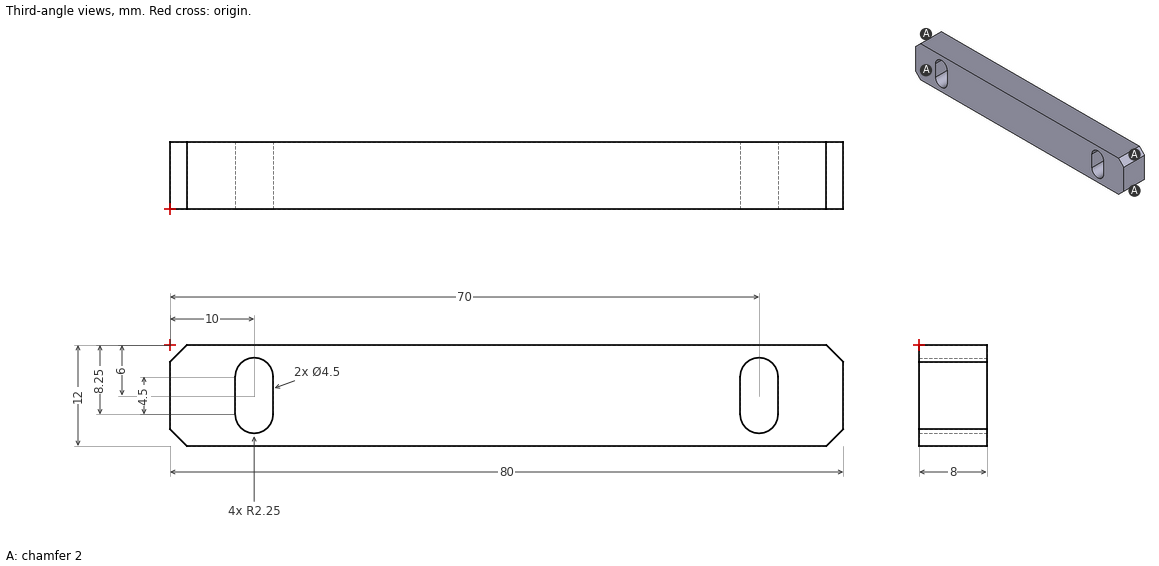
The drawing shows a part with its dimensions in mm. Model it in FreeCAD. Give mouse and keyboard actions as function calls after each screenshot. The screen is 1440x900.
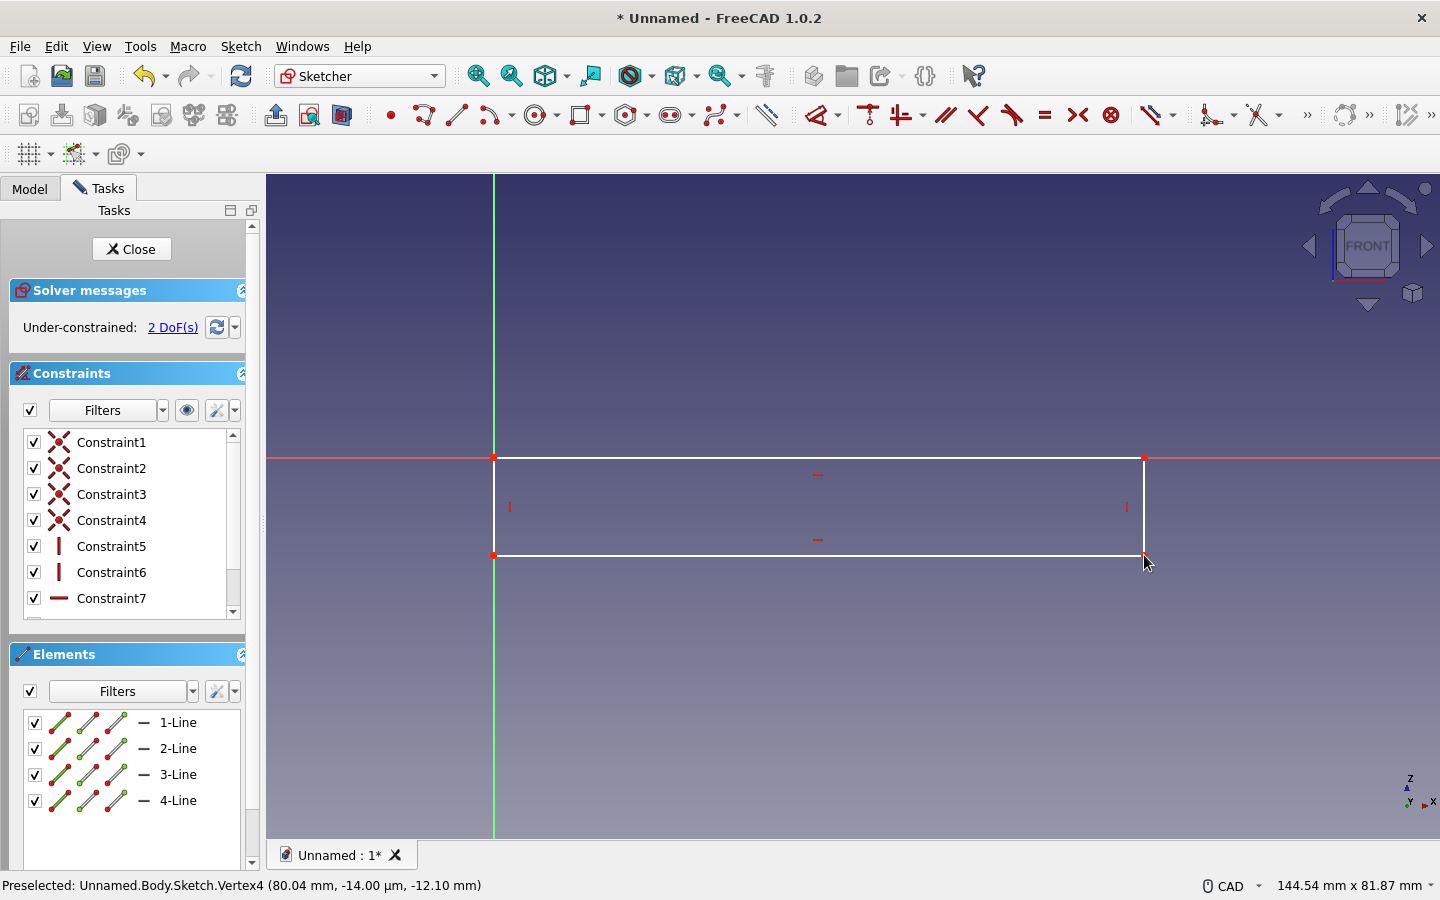
key(d)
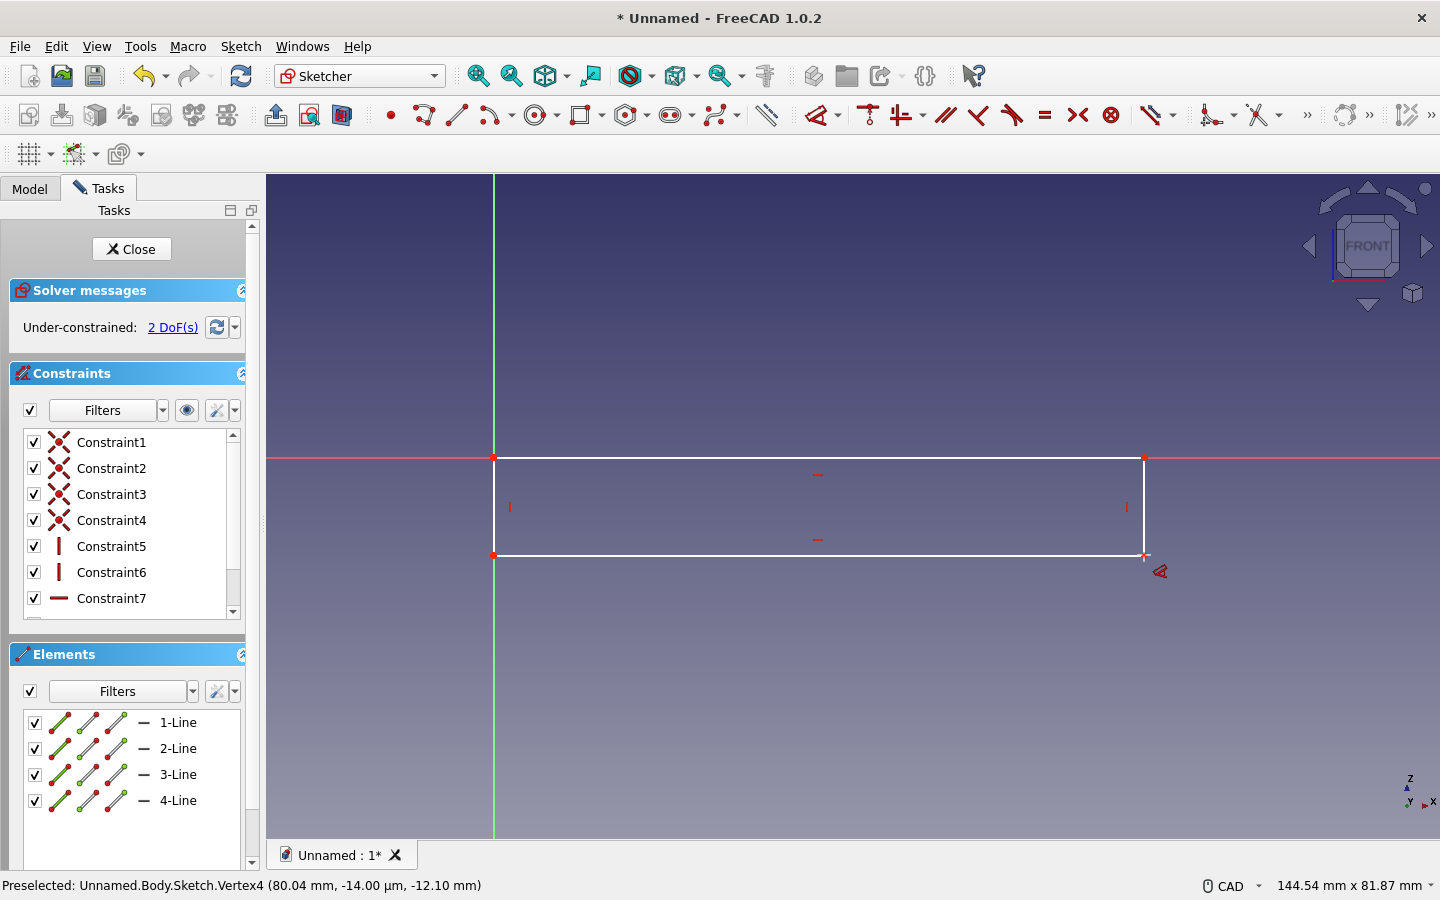
click(494, 487)
click(460, 507)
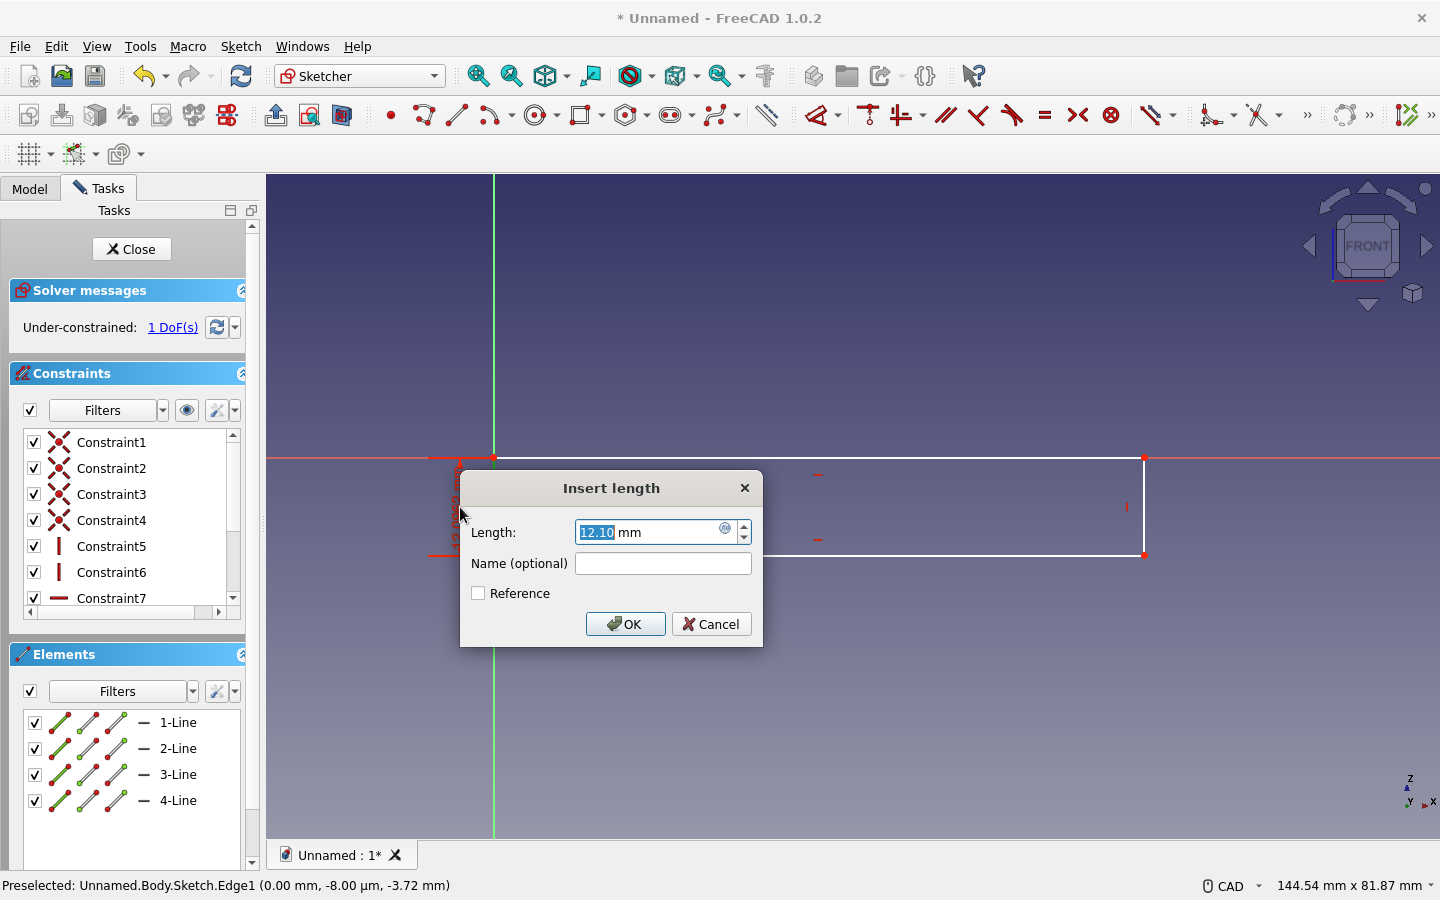
text(12)
key(Return)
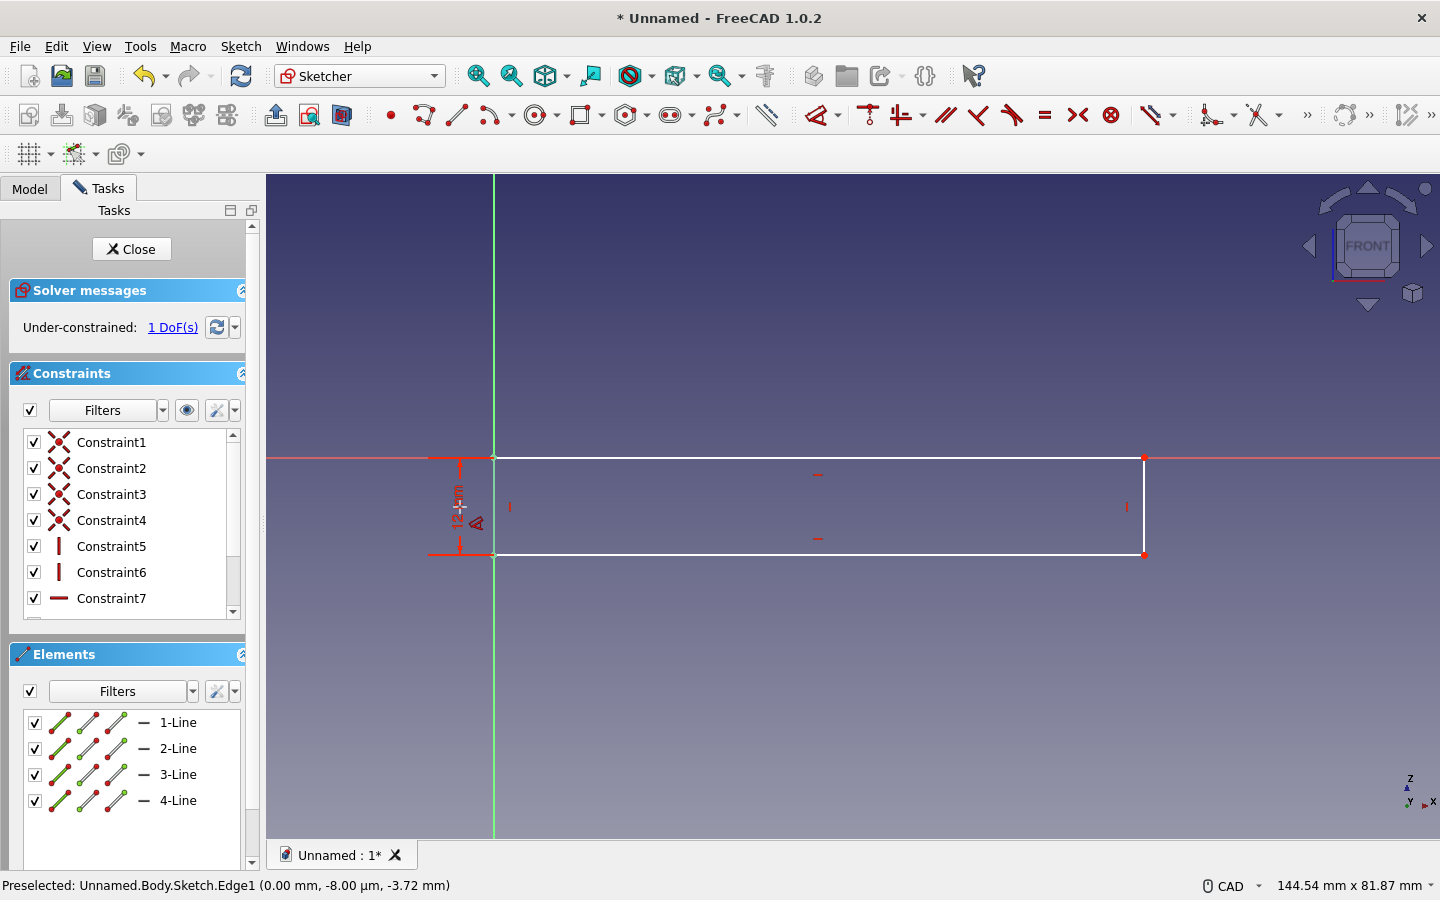
click(689, 555)
click(819, 589)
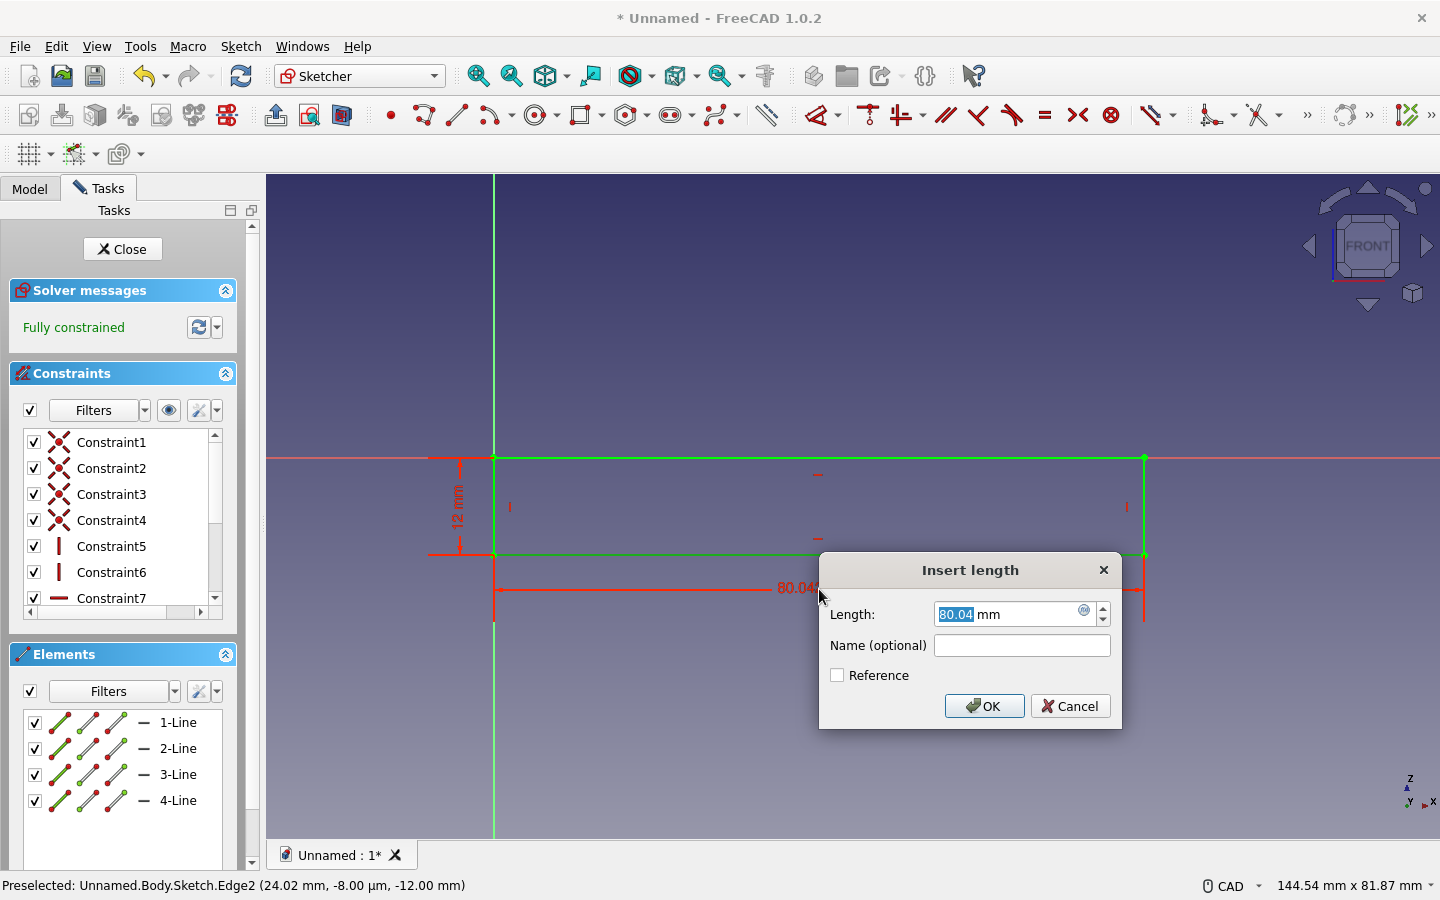
text(80)
key(Return)
key(Escape)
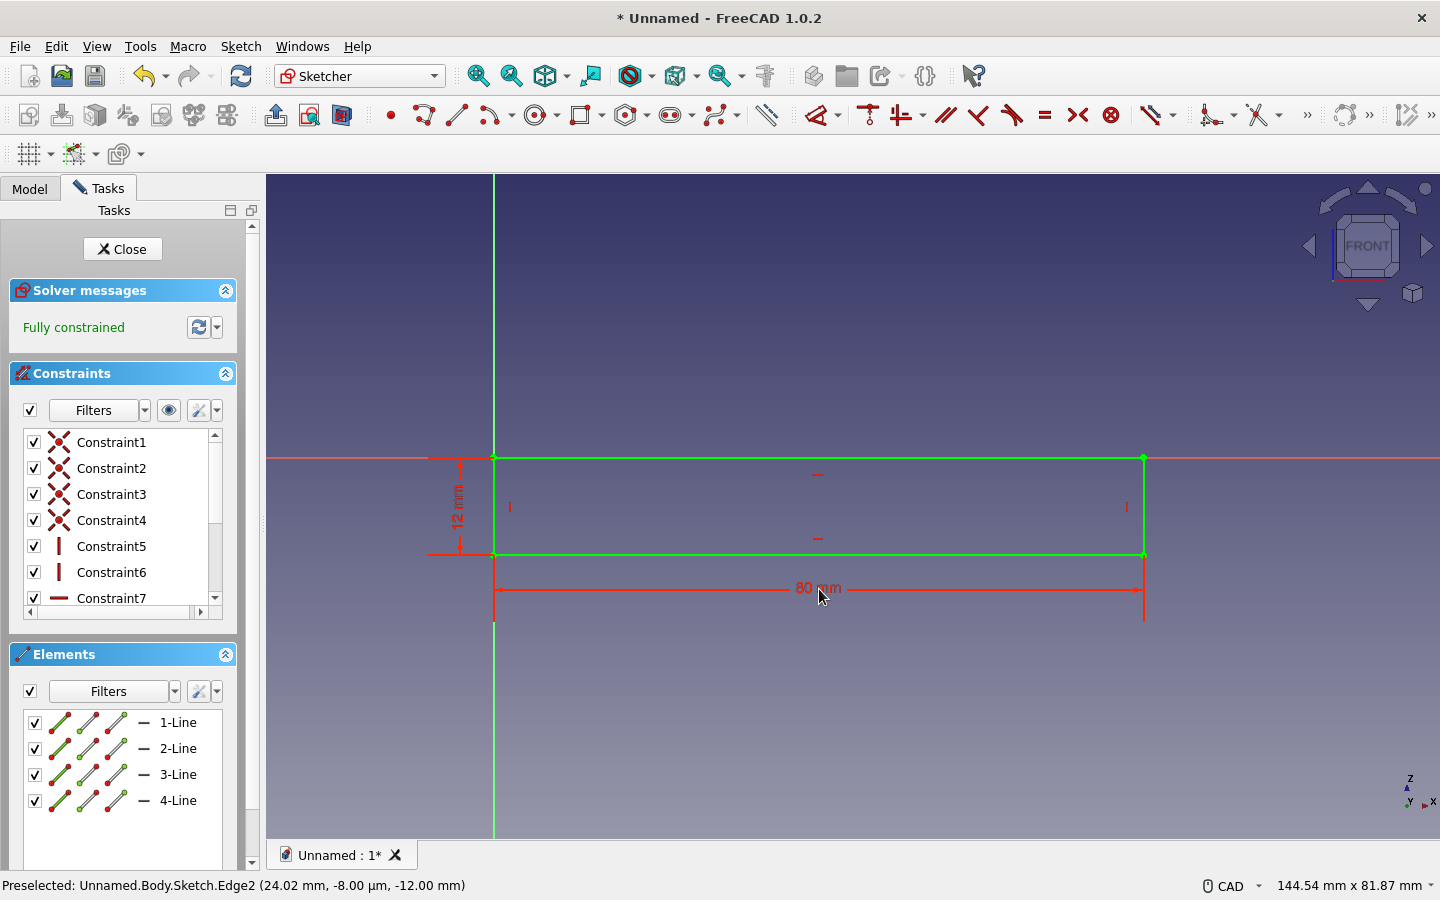
click(123, 249)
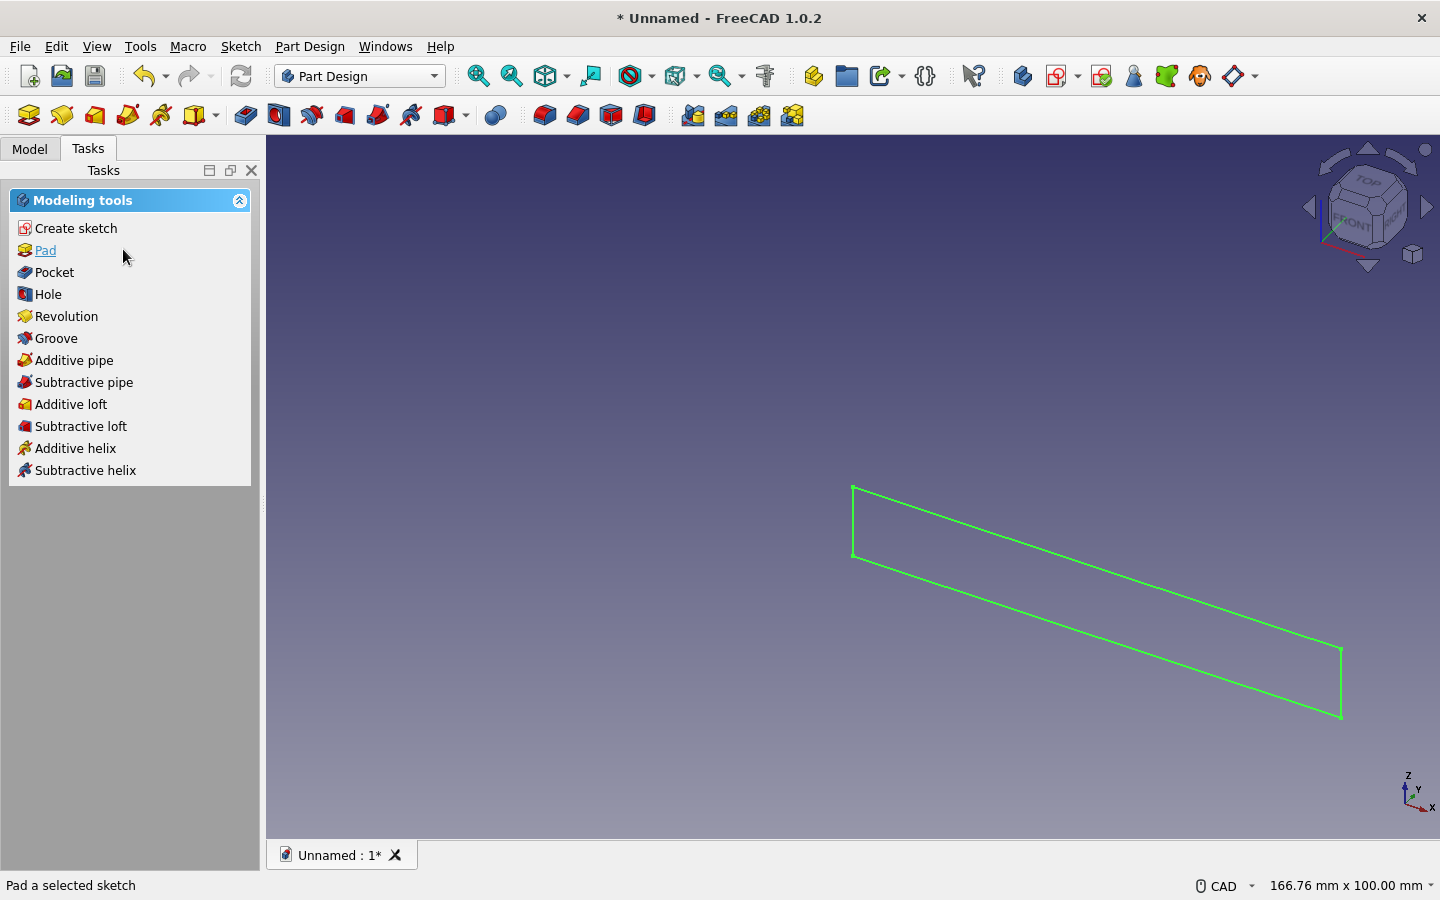
click(29, 116)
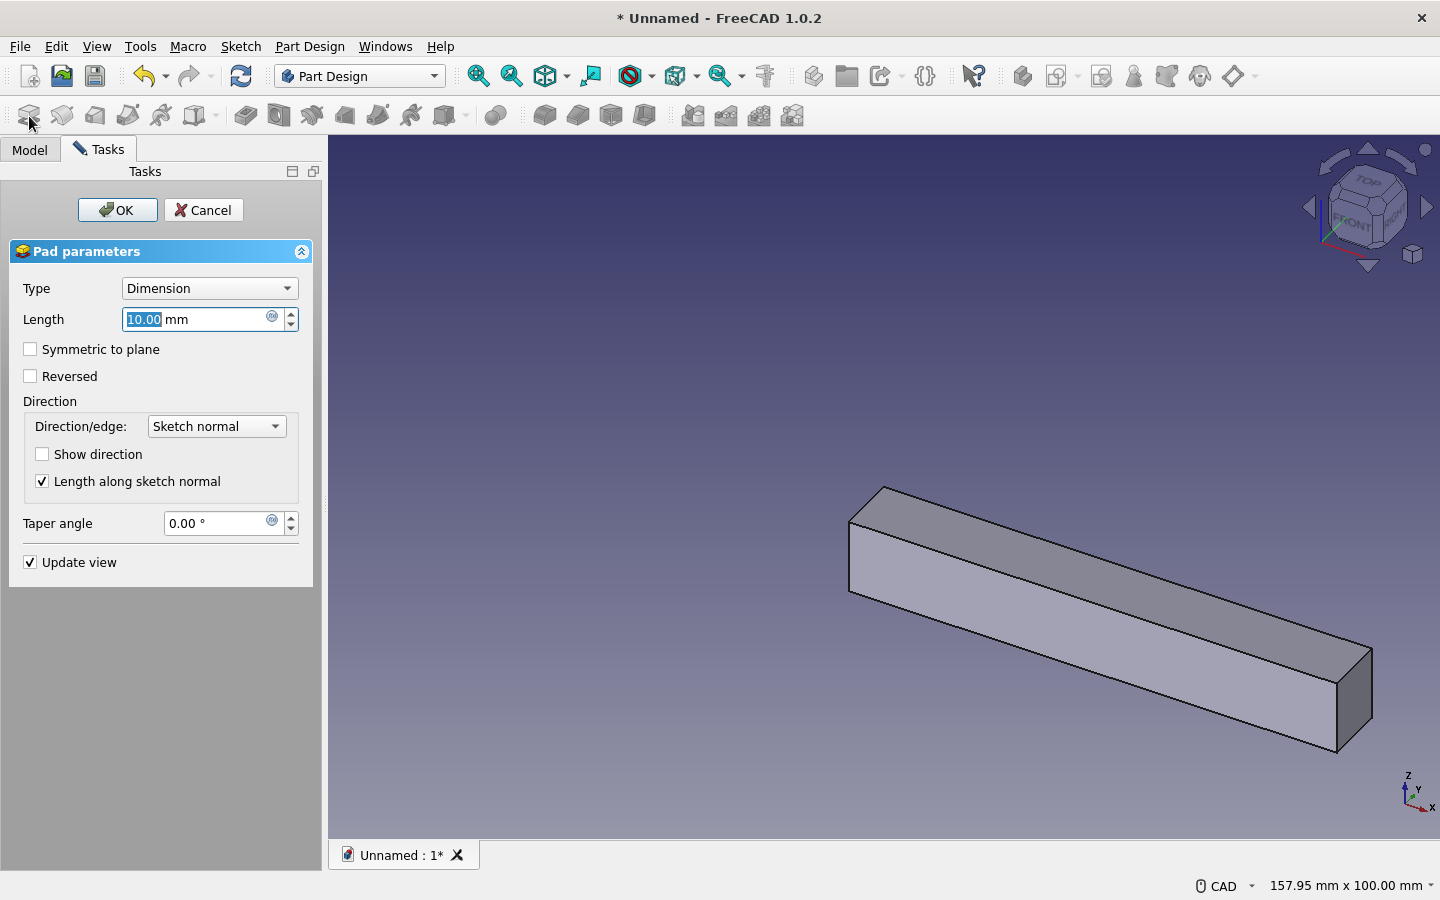
text(8)
key(Tab)